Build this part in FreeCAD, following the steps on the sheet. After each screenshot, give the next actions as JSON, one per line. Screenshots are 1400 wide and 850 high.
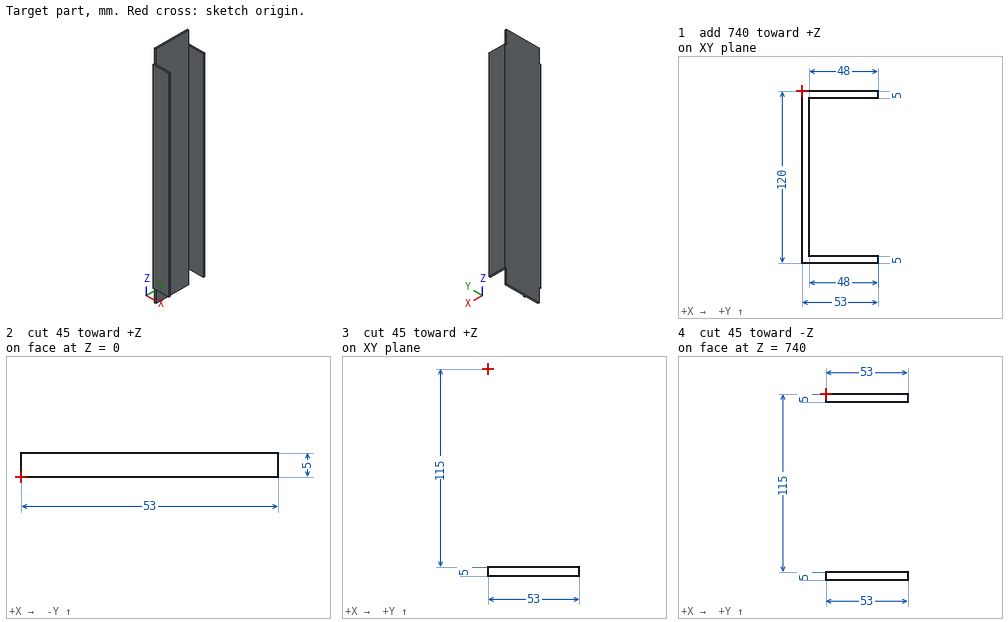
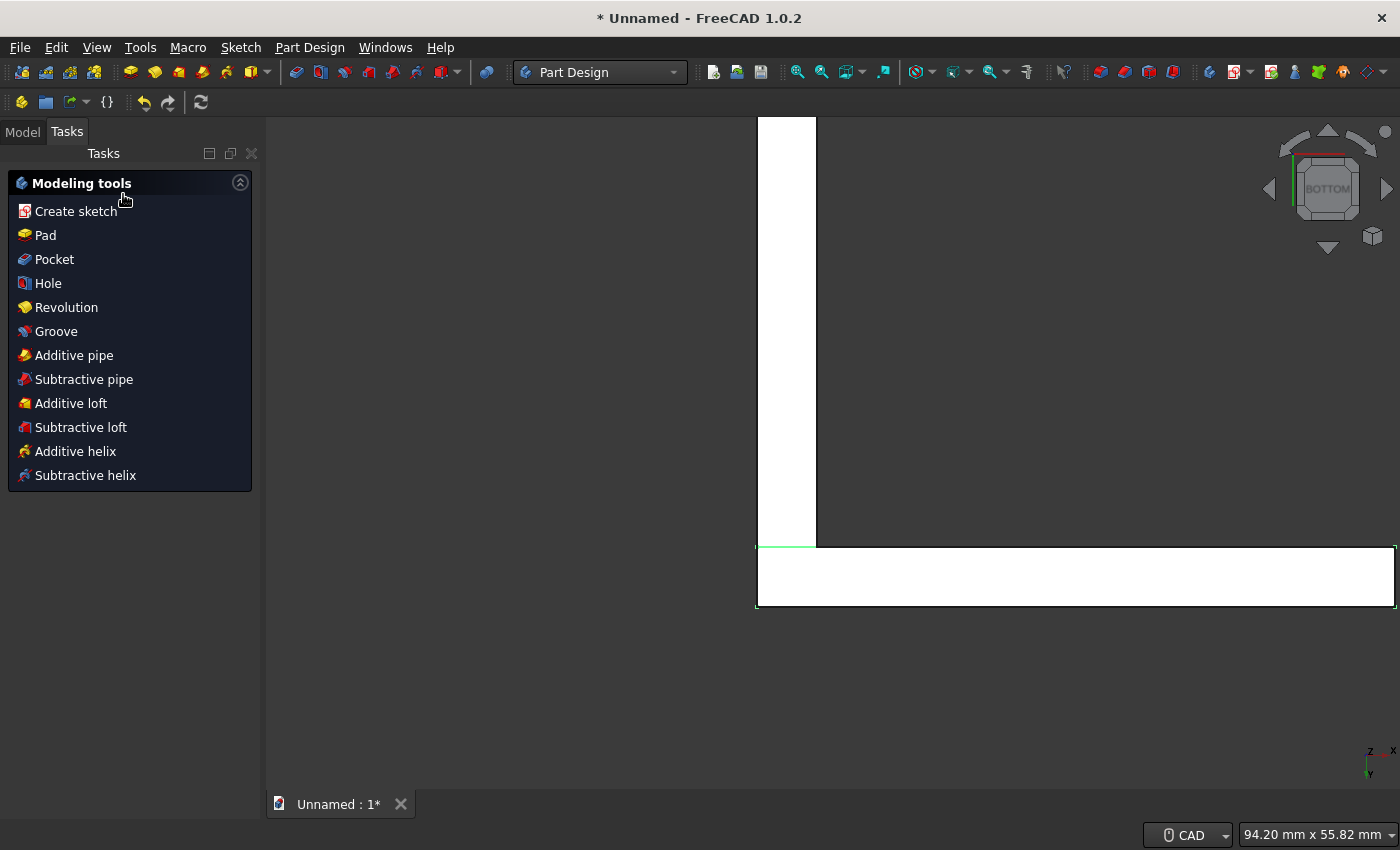
{"action": "left_click", "coordinate": [298, 72]}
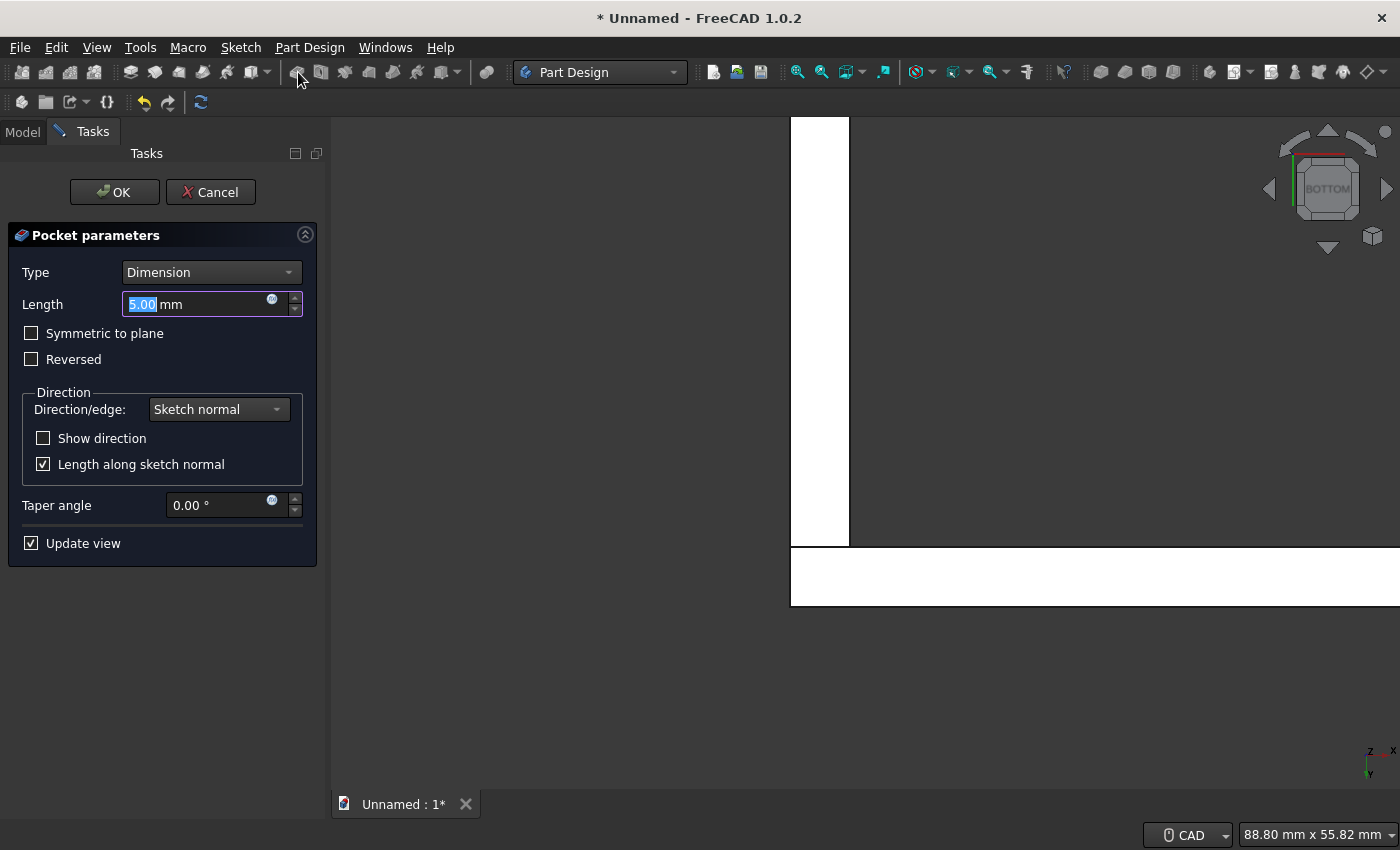
{"action": "type", "text": "45"}
{"action": "key", "text": "Tab"}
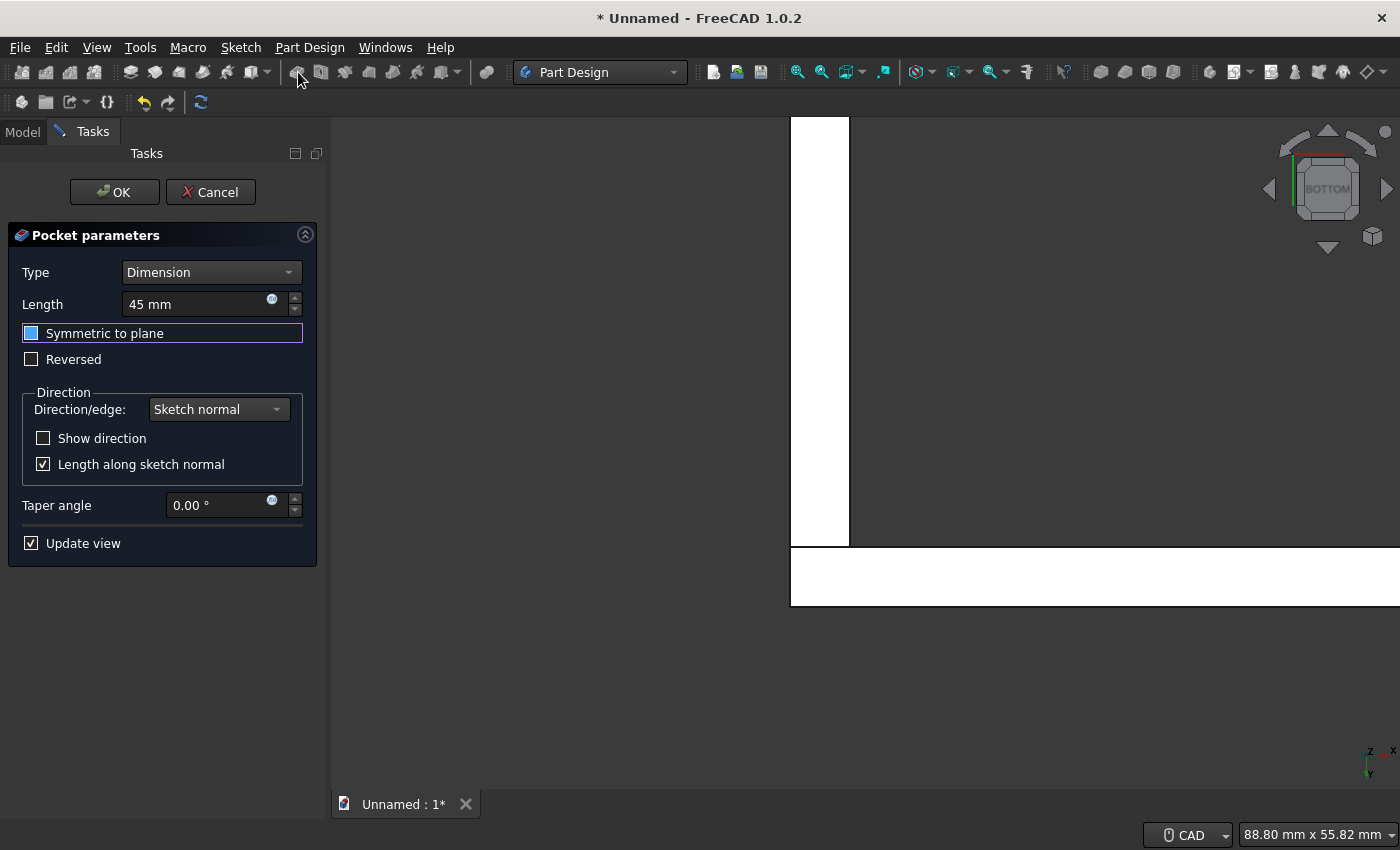
{"action": "left_click", "coordinate": [115, 192]}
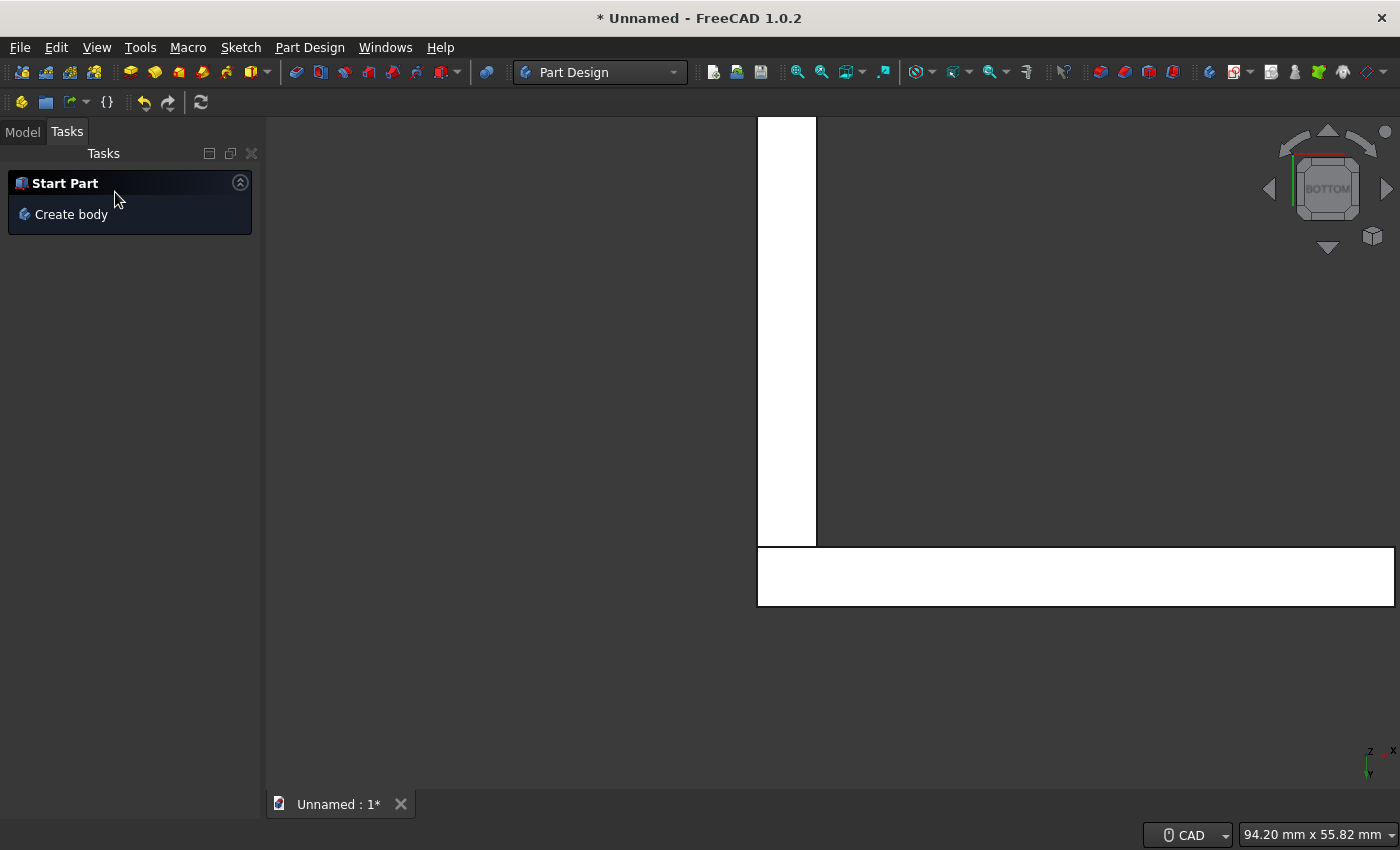
{"action": "left_click", "coordinate": [798, 72]}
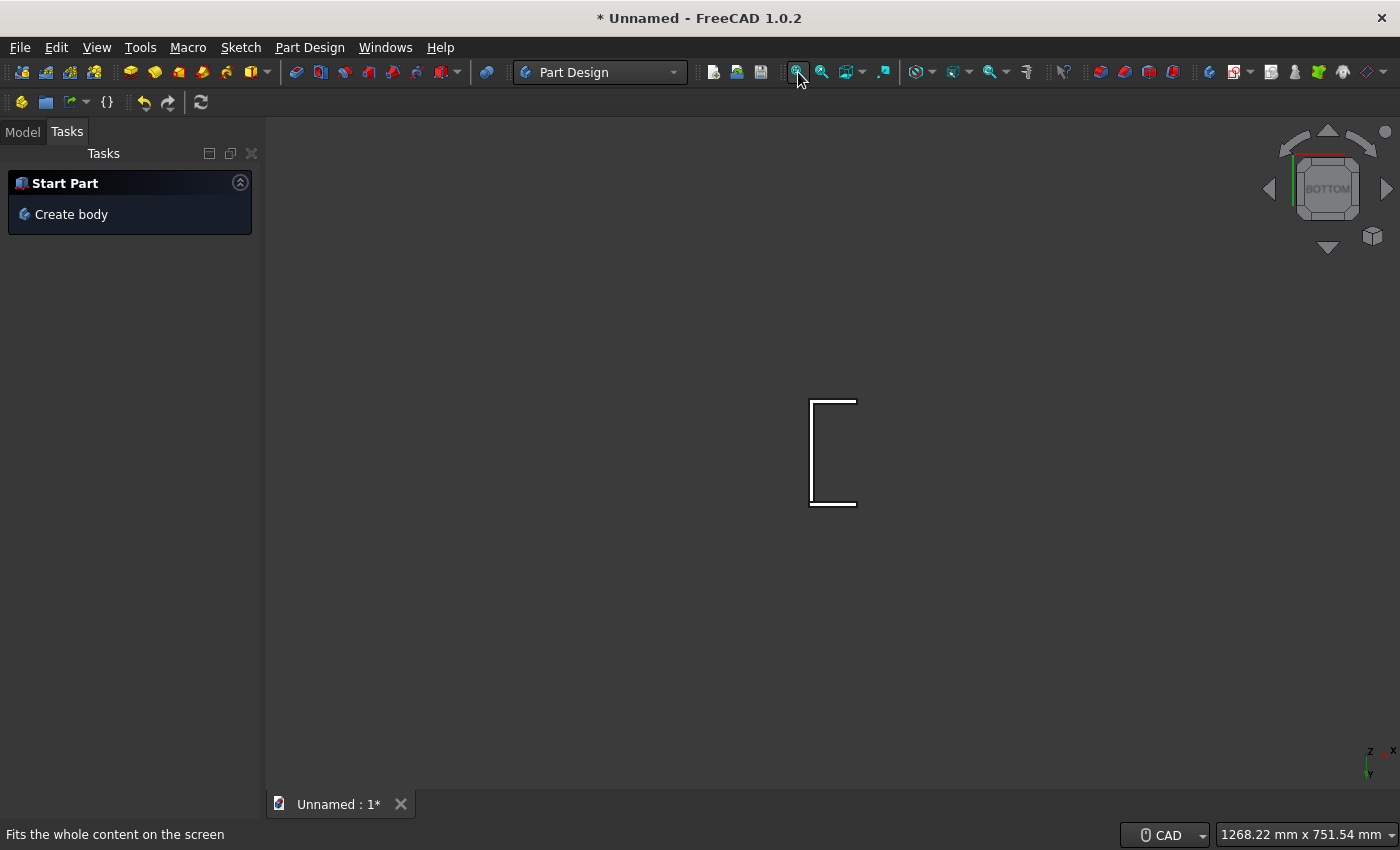
{"action": "left_click", "coordinate": [1234, 72]}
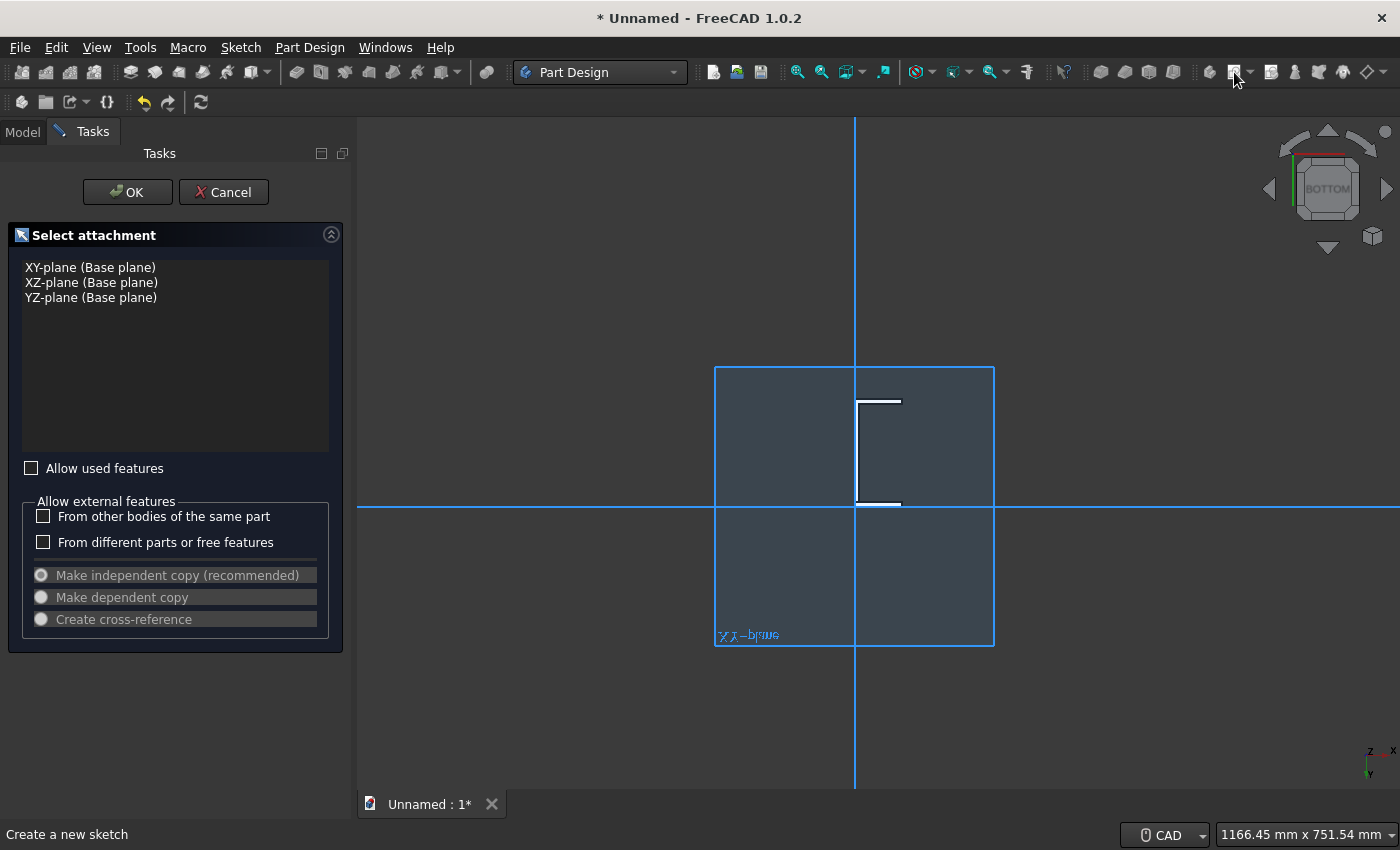
{"action": "left_click", "coordinate": [82, 268]}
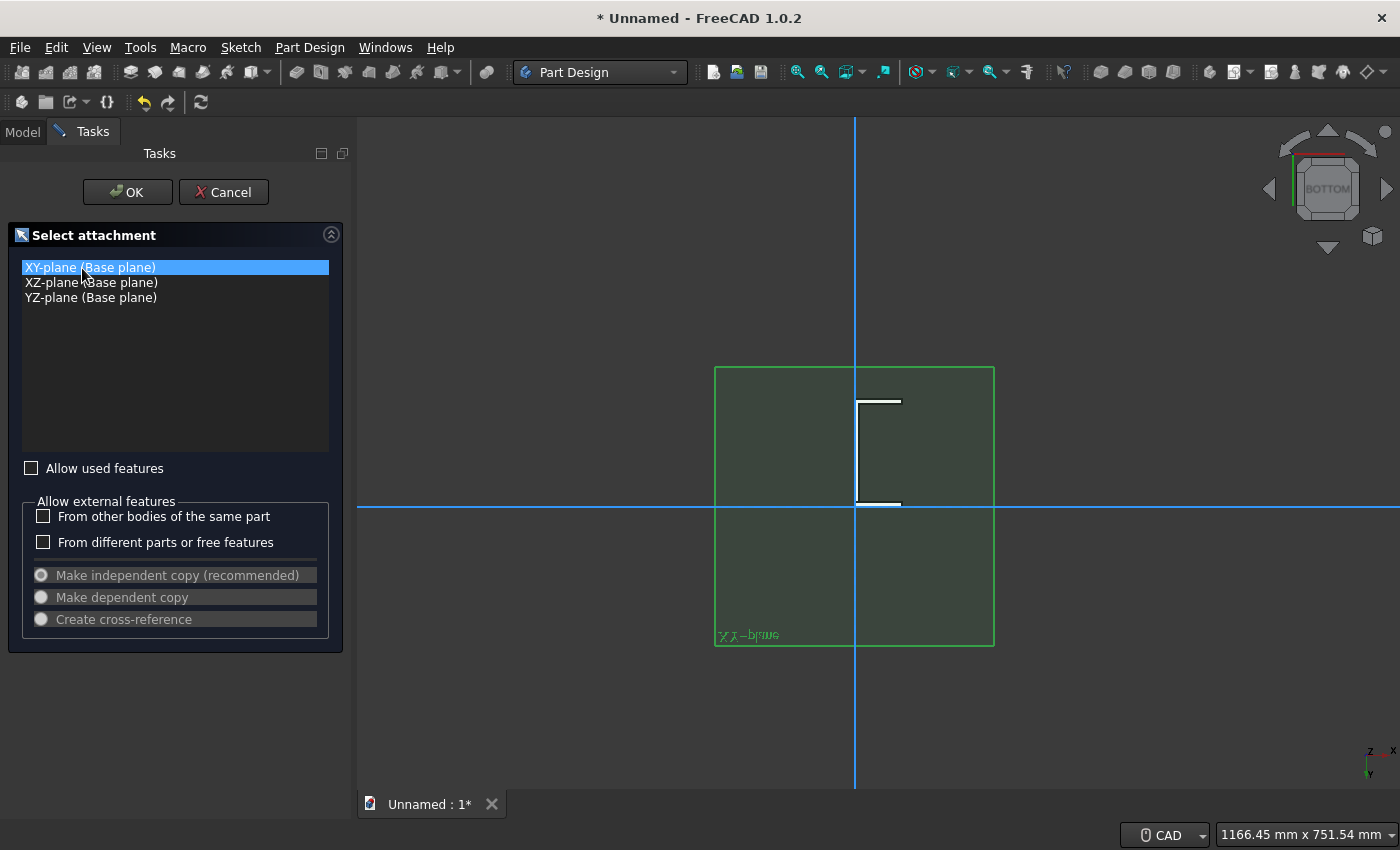
{"action": "left_click", "coordinate": [128, 192]}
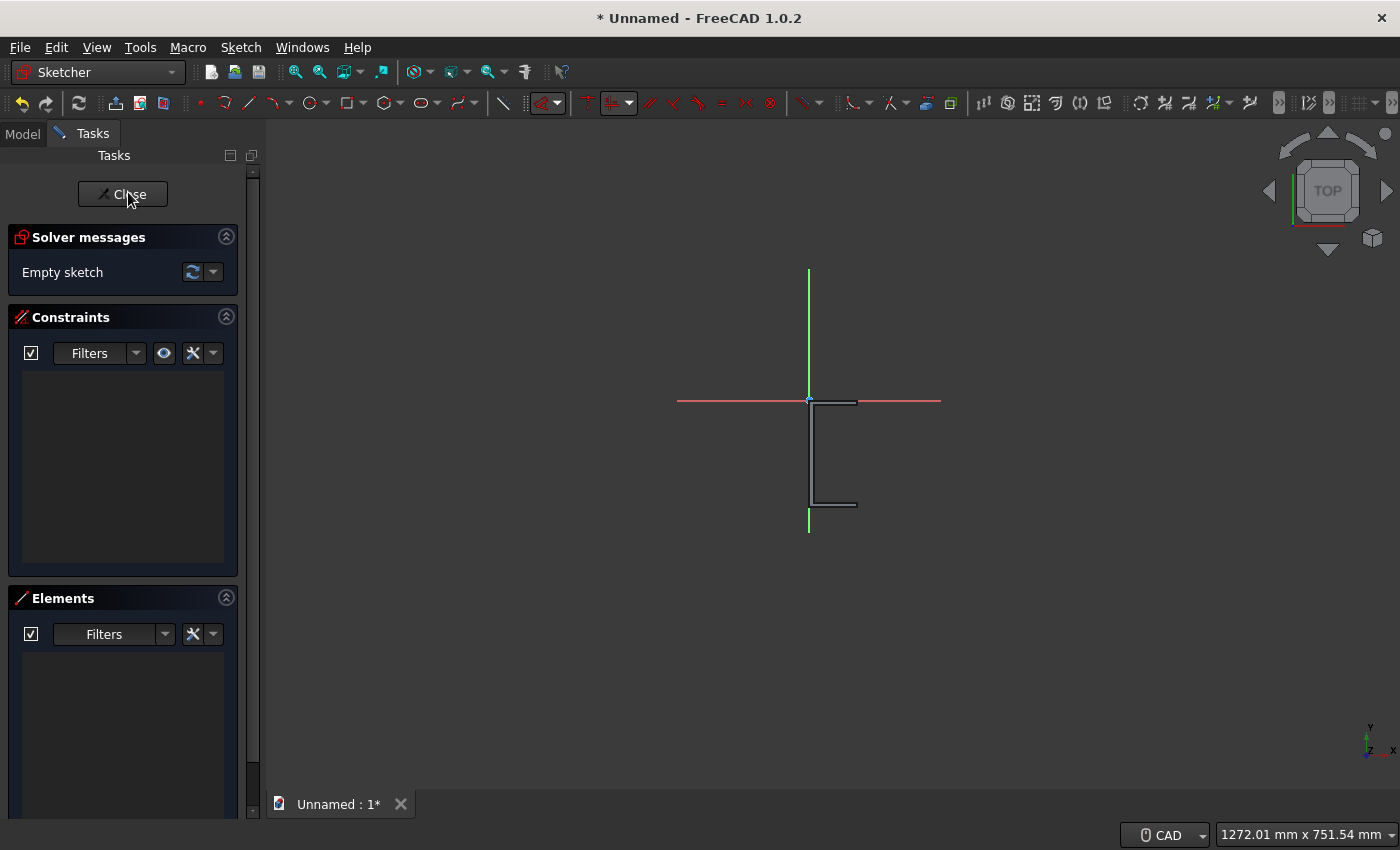
{"action": "left_click", "coordinate": [164, 104]}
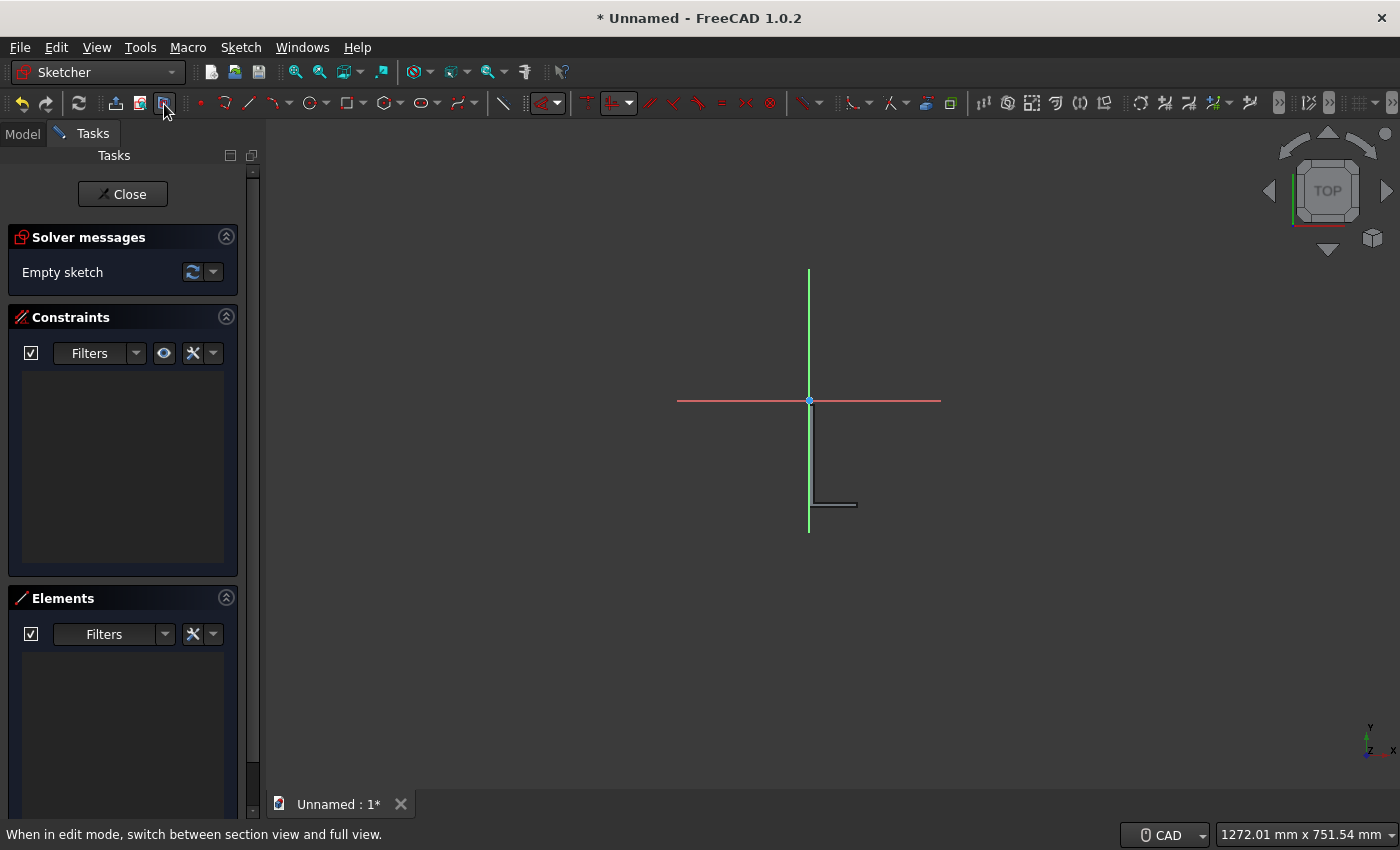
{"action": "scroll", "coordinate": [855, 454], "scroll_direction": "up", "scroll_amount": 7}